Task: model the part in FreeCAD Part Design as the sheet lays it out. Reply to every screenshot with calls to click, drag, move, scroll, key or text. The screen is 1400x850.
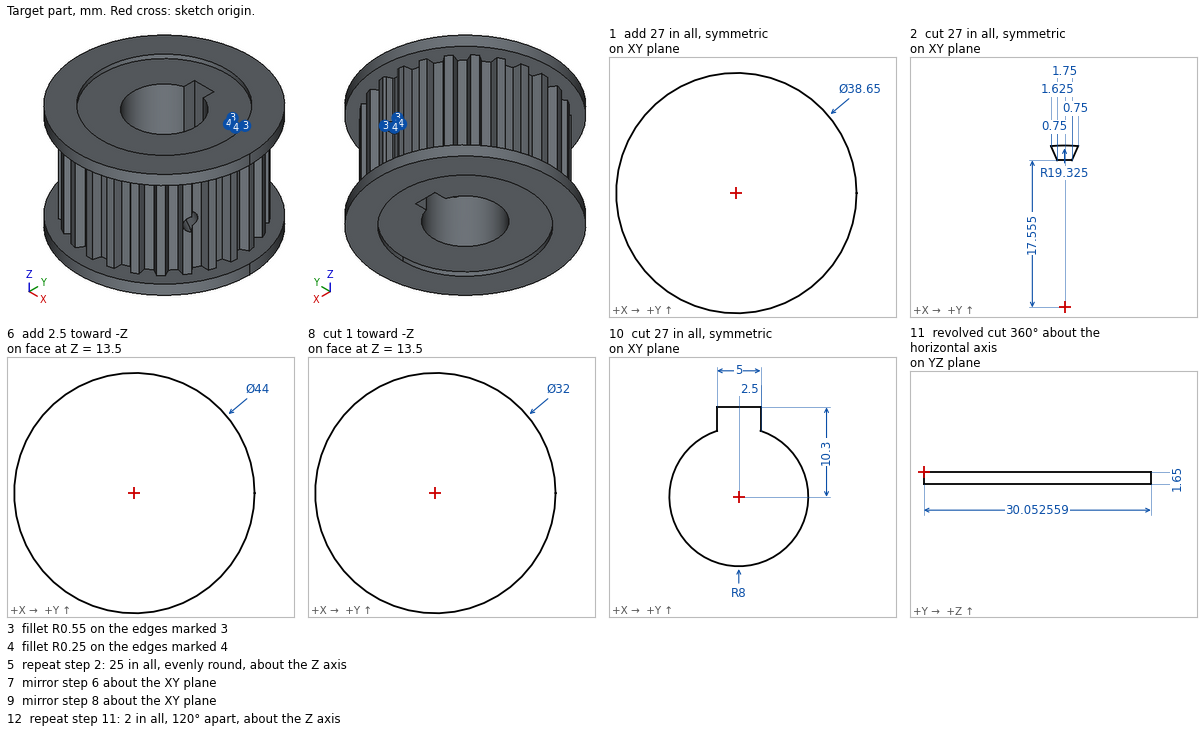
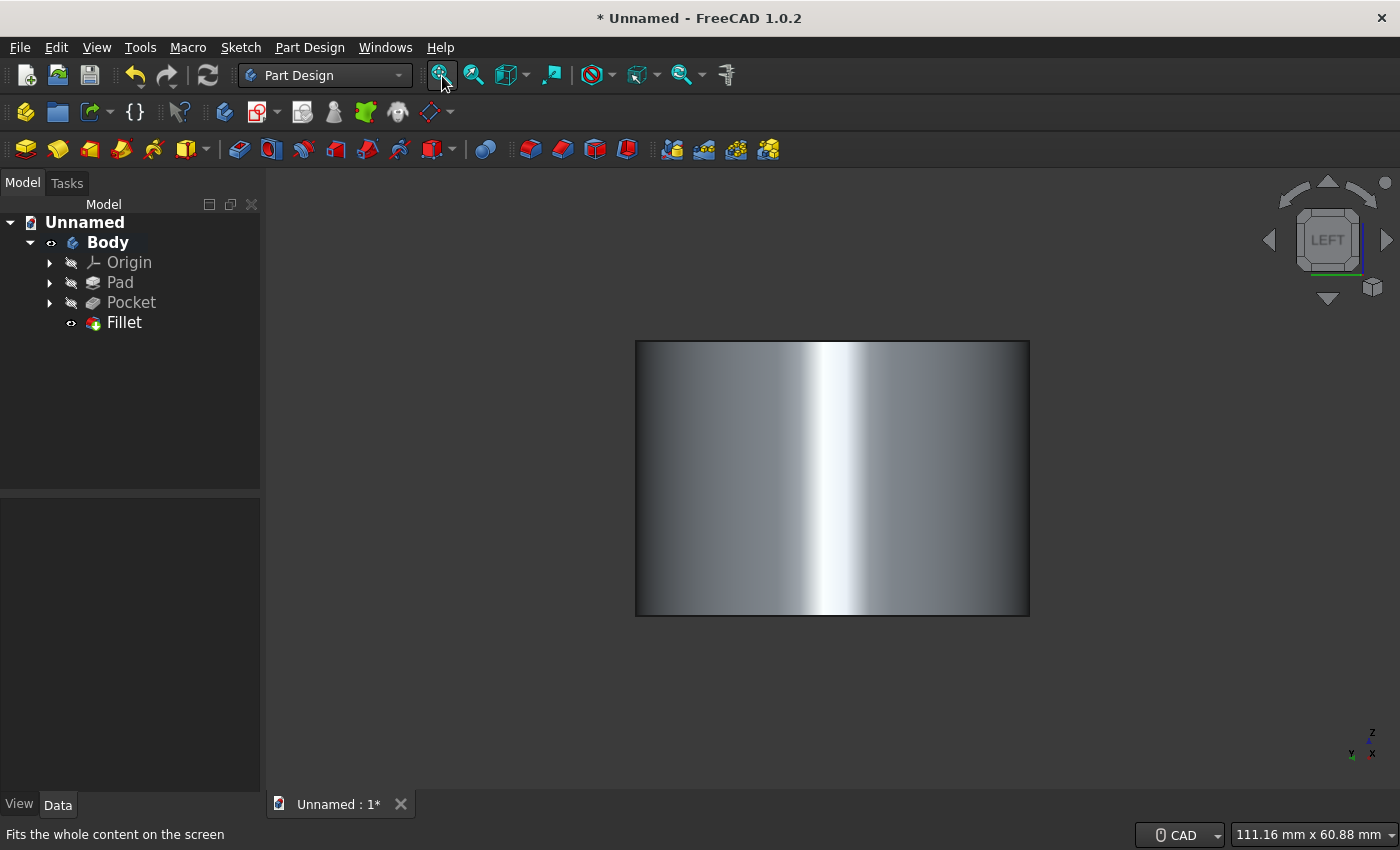
key(v)
key(3)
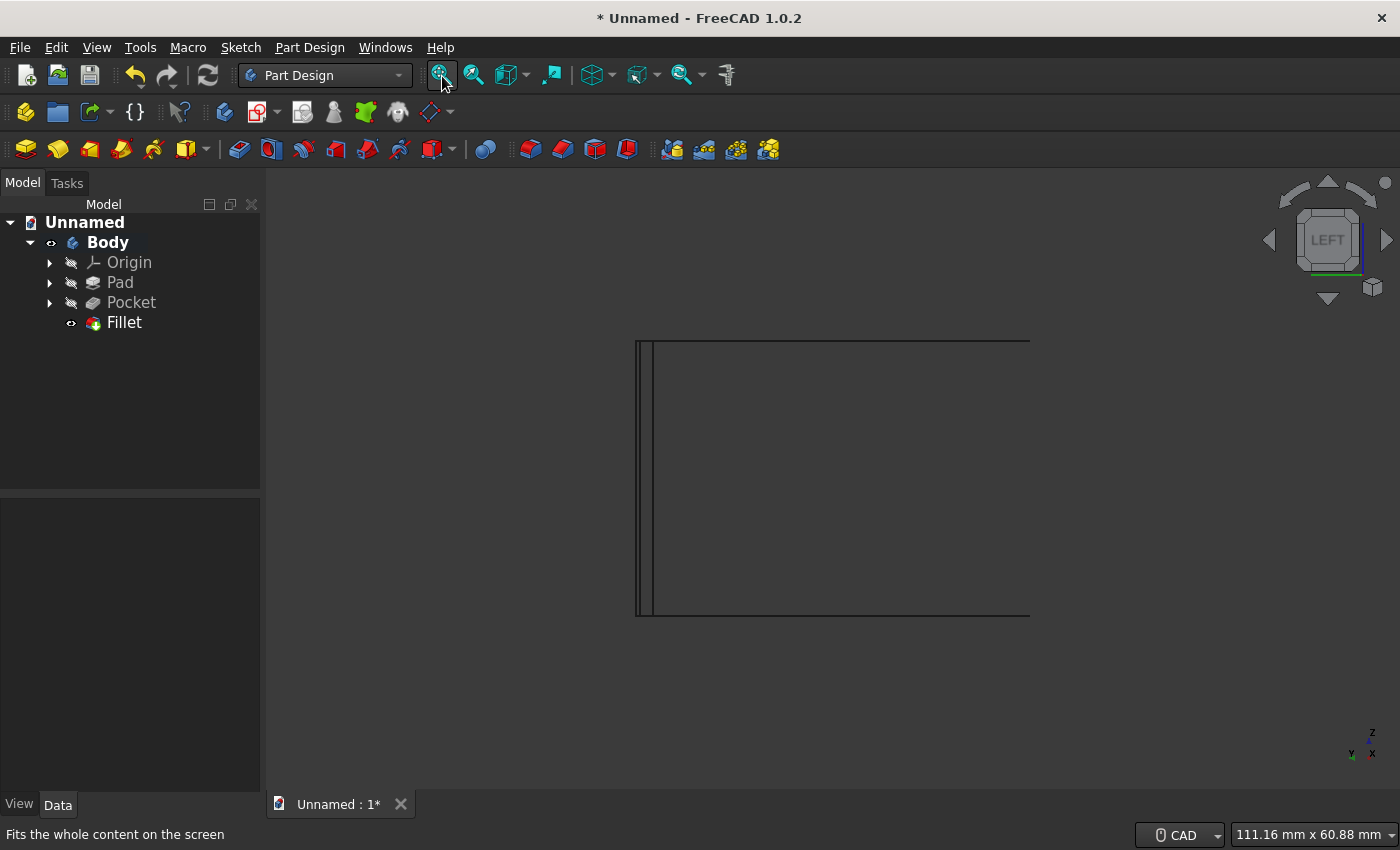
key(0)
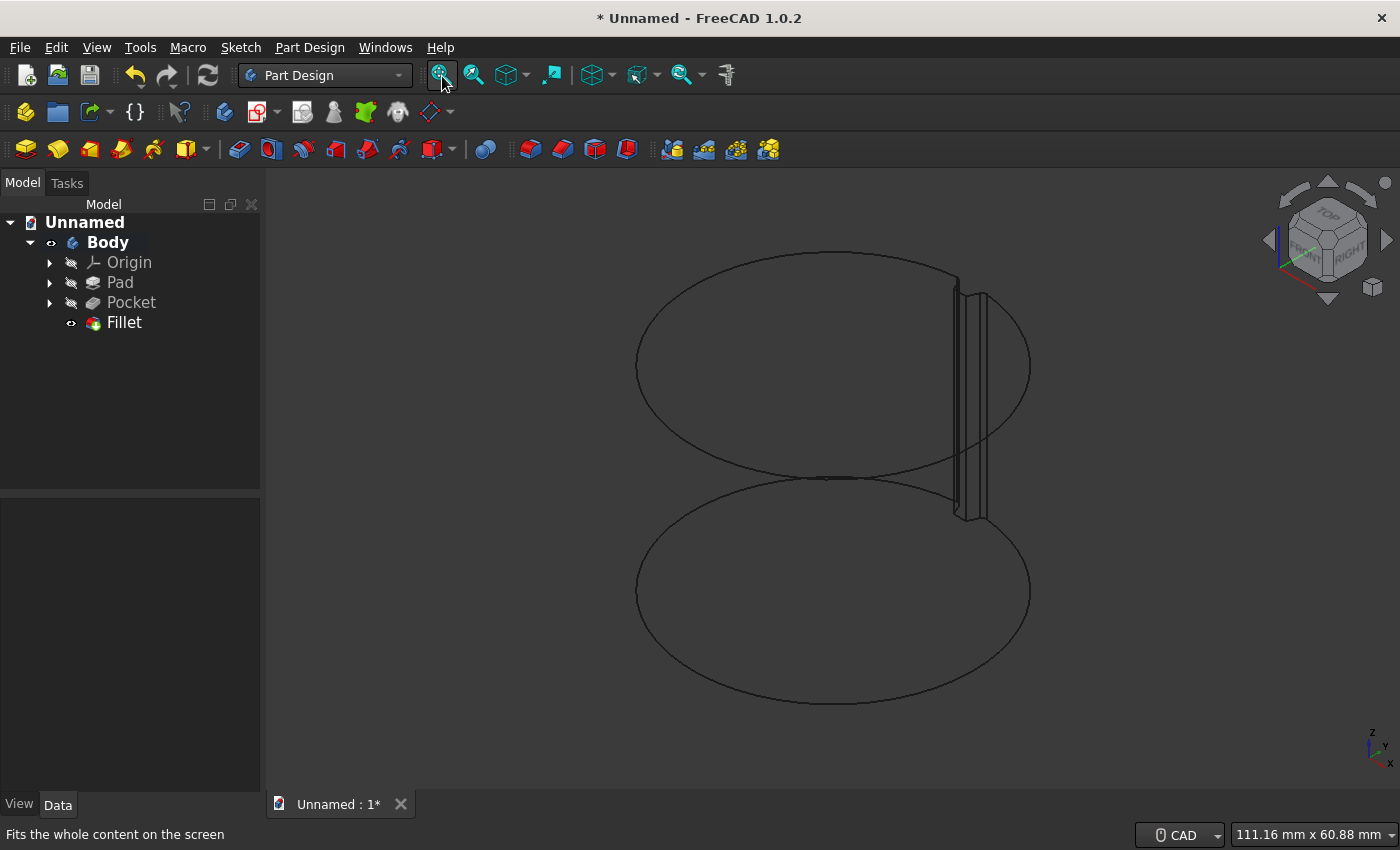
click(954, 401)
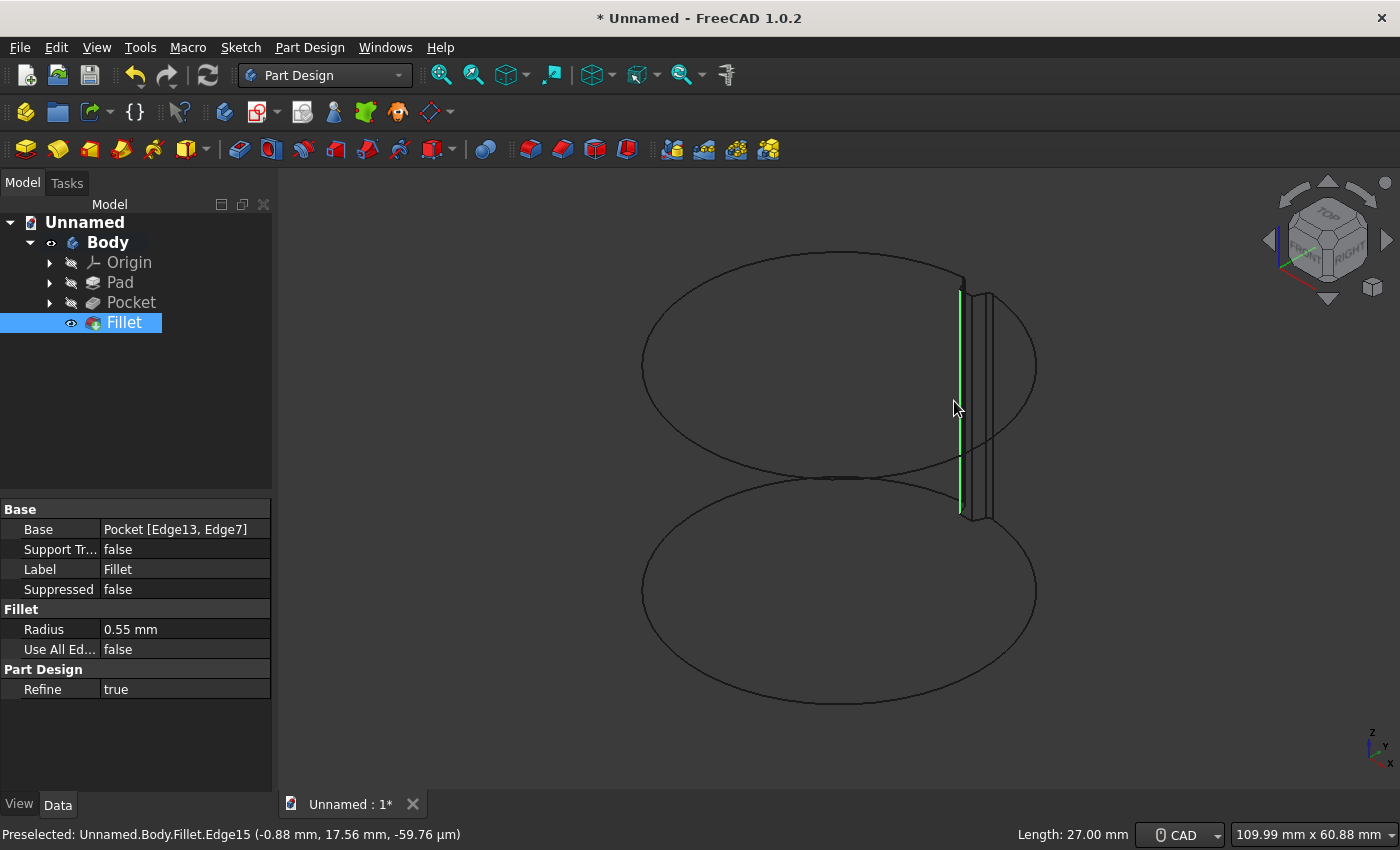
click(972, 408, ctrl)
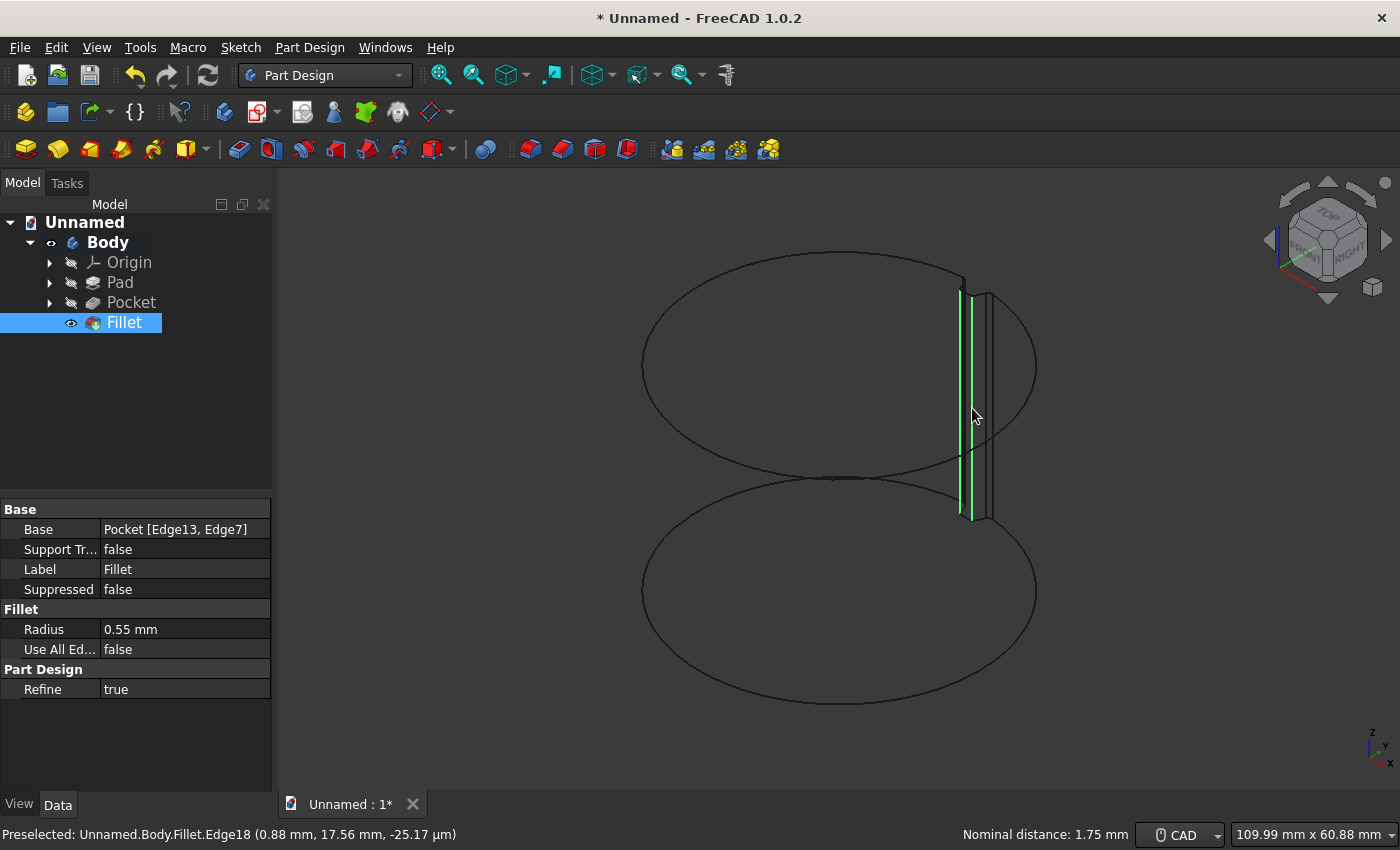
key(v)
key(1)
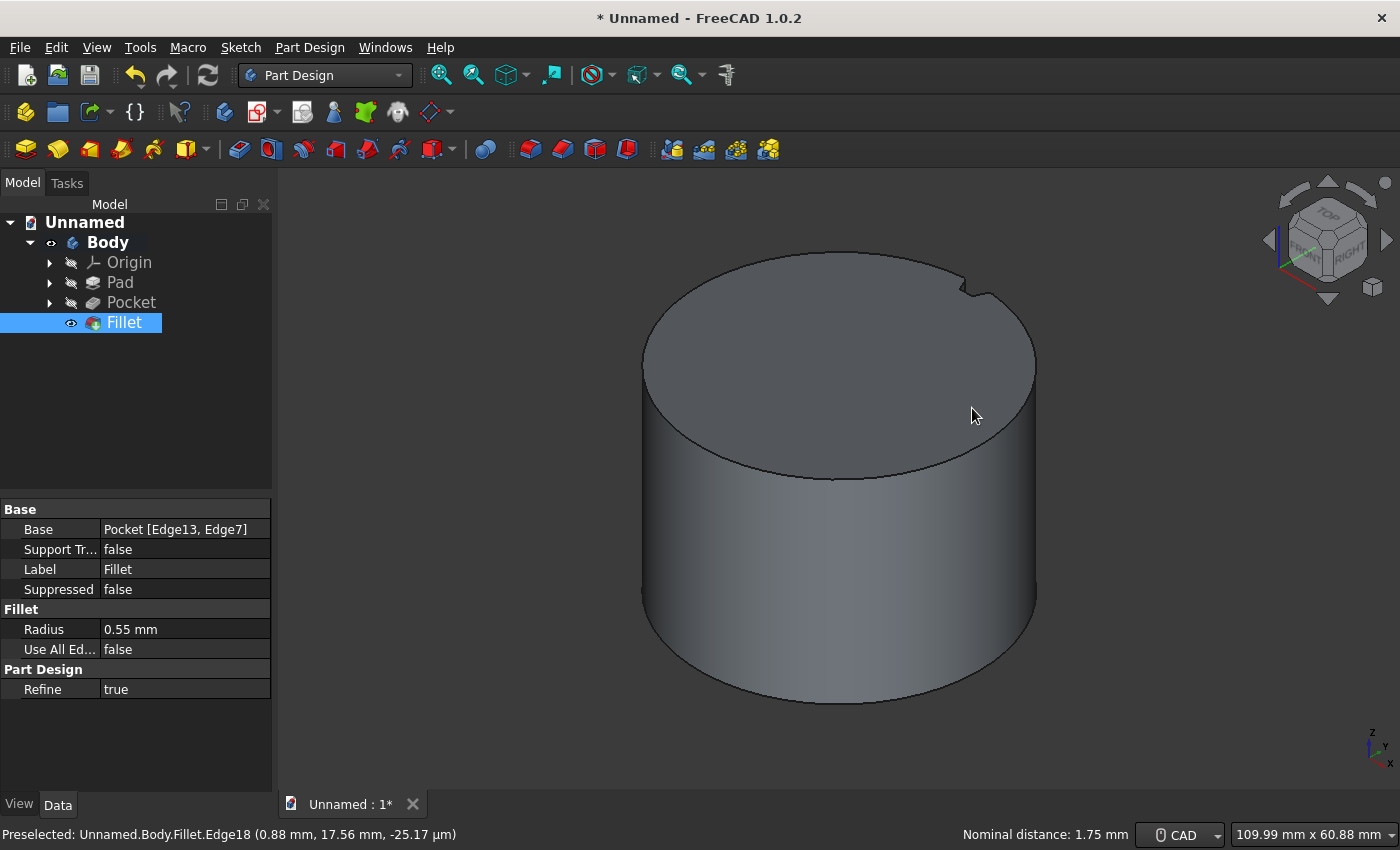
click(532, 150)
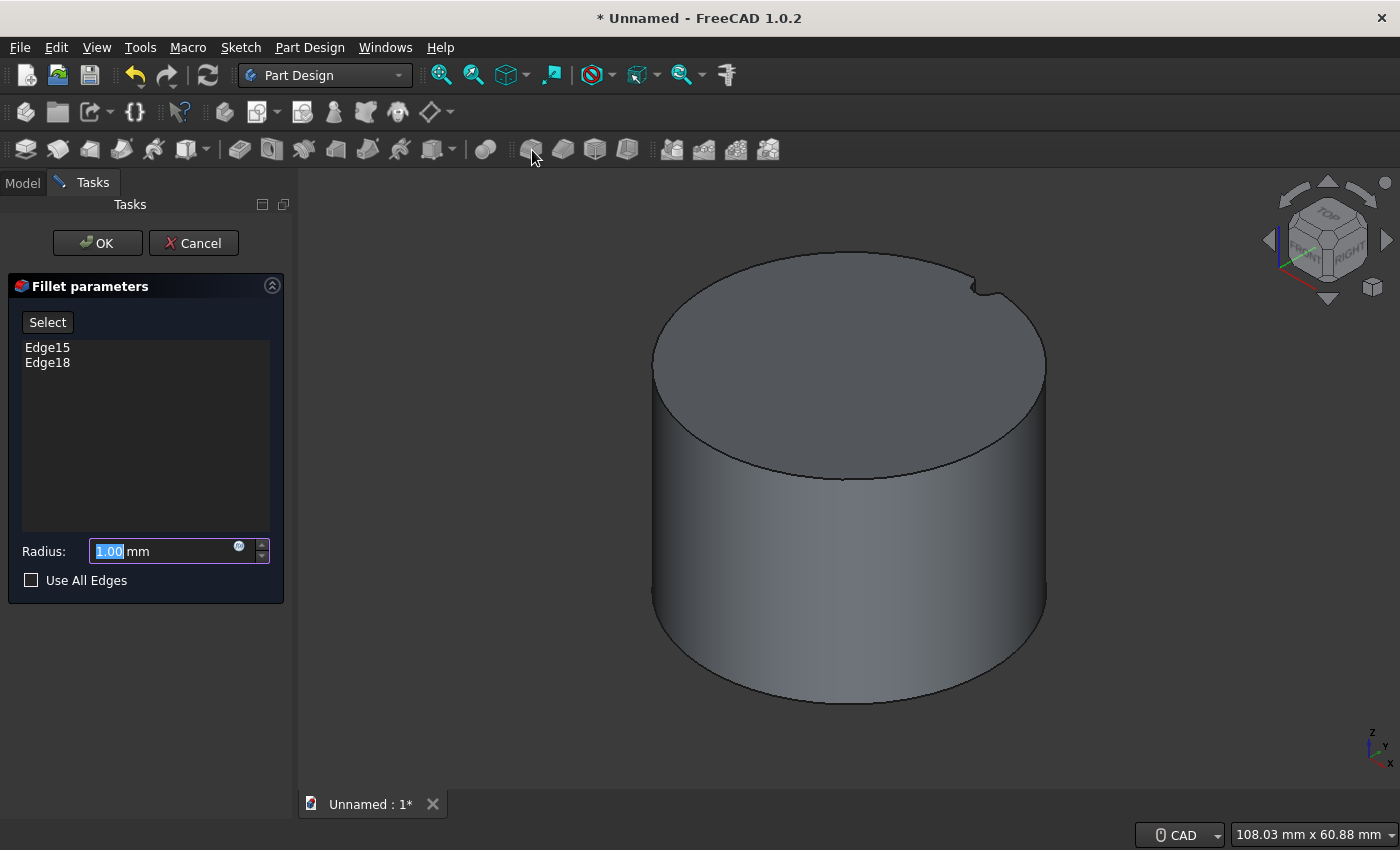
text(0.25)
key(Tab)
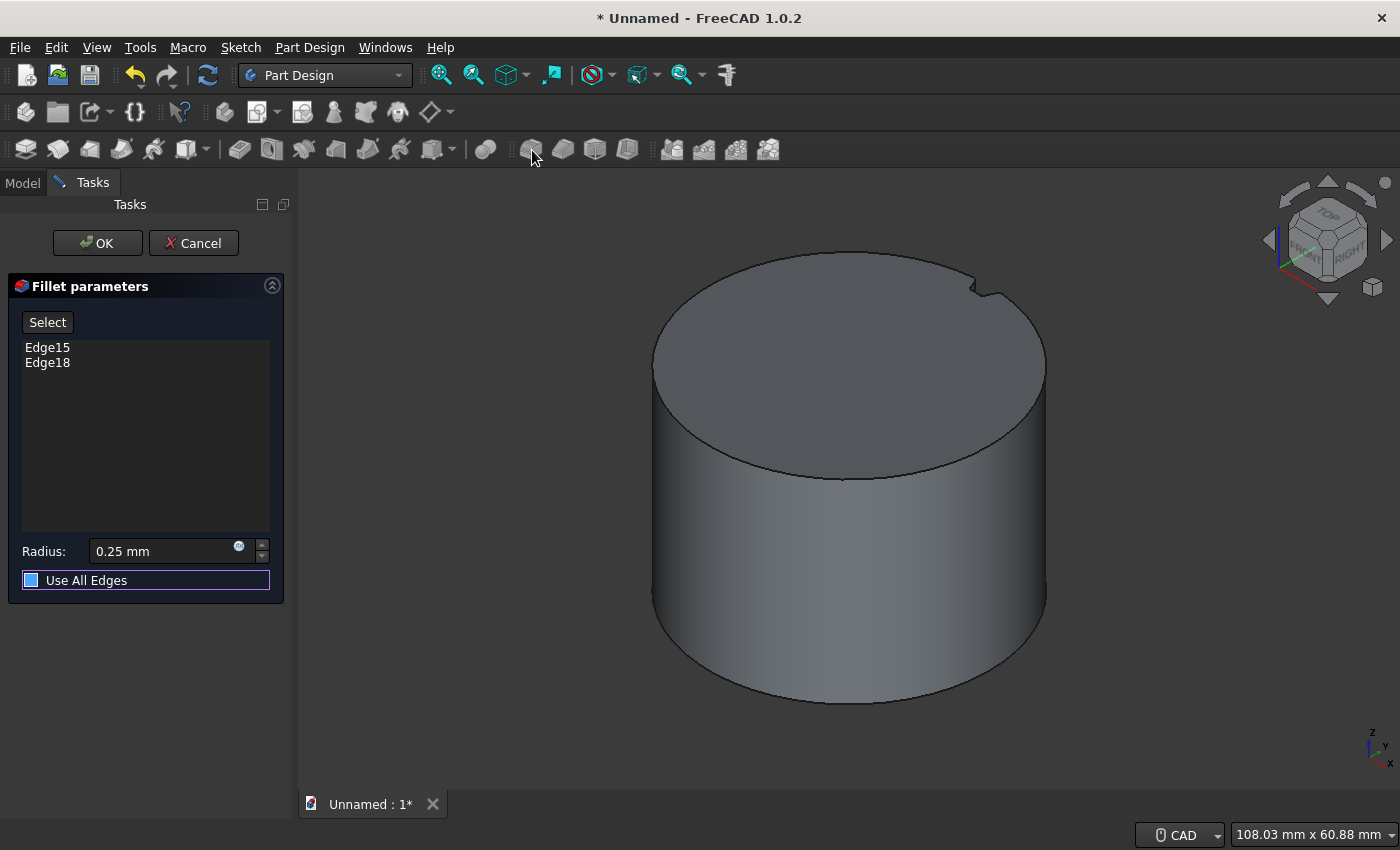
click(98, 243)